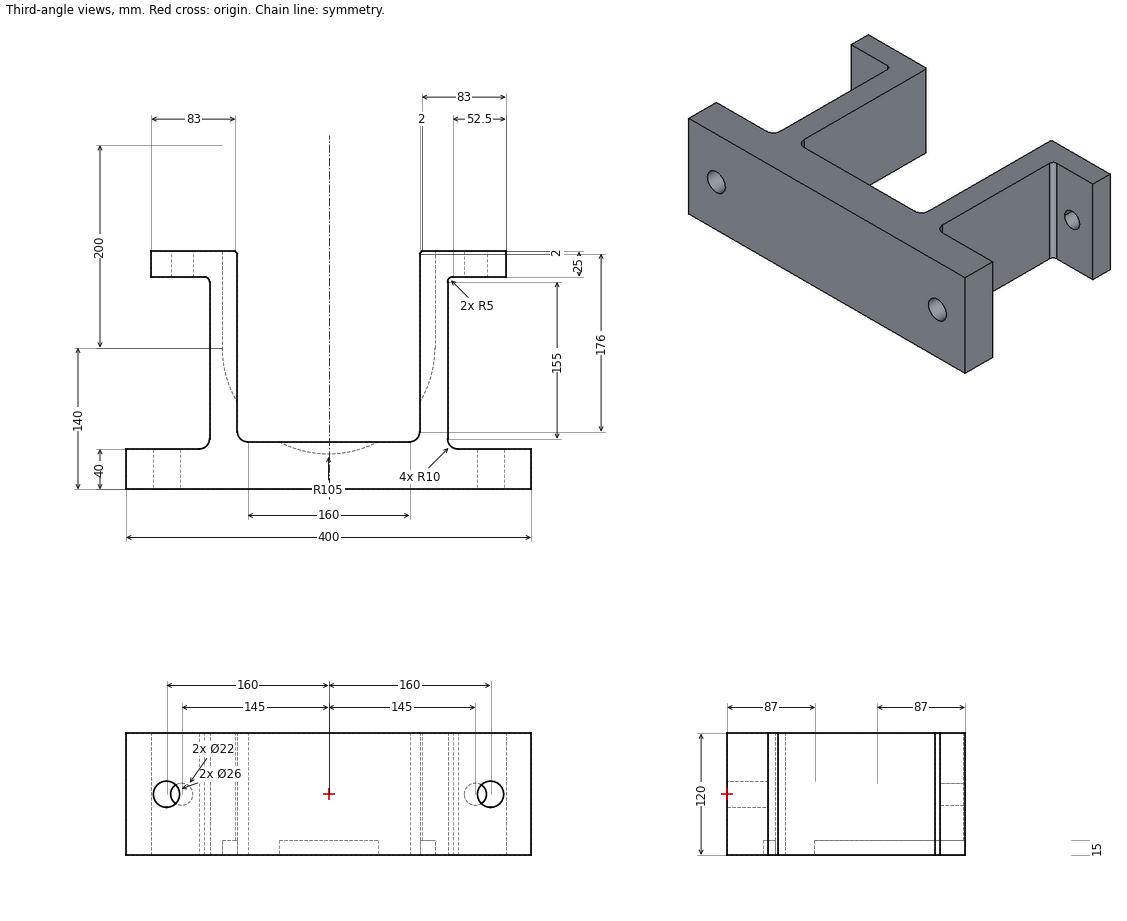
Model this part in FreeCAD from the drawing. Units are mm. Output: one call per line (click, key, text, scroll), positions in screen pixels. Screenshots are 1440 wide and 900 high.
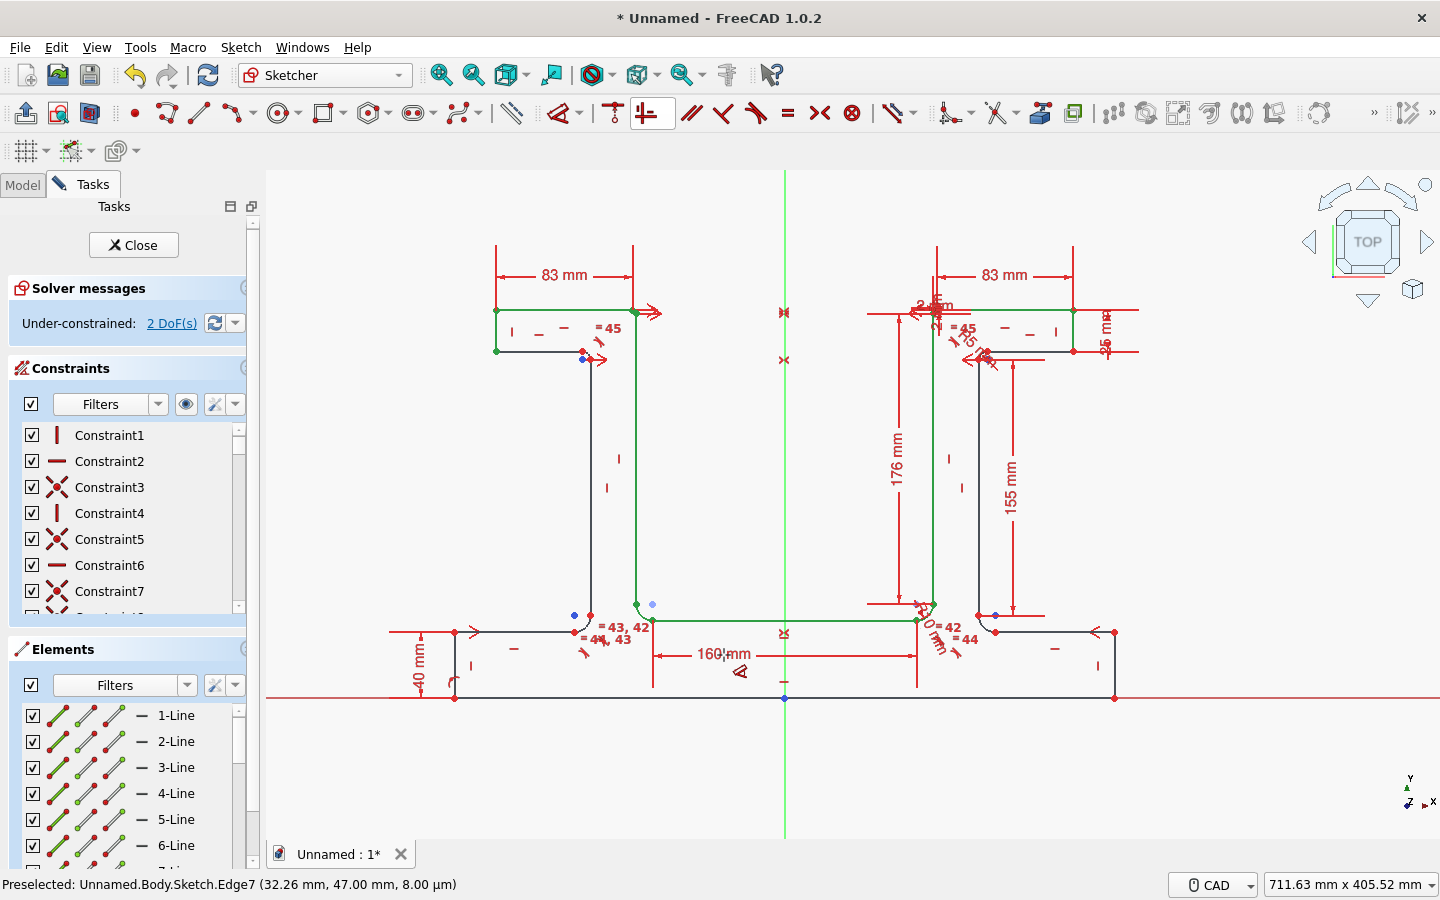
click(653, 698)
click(633, 732)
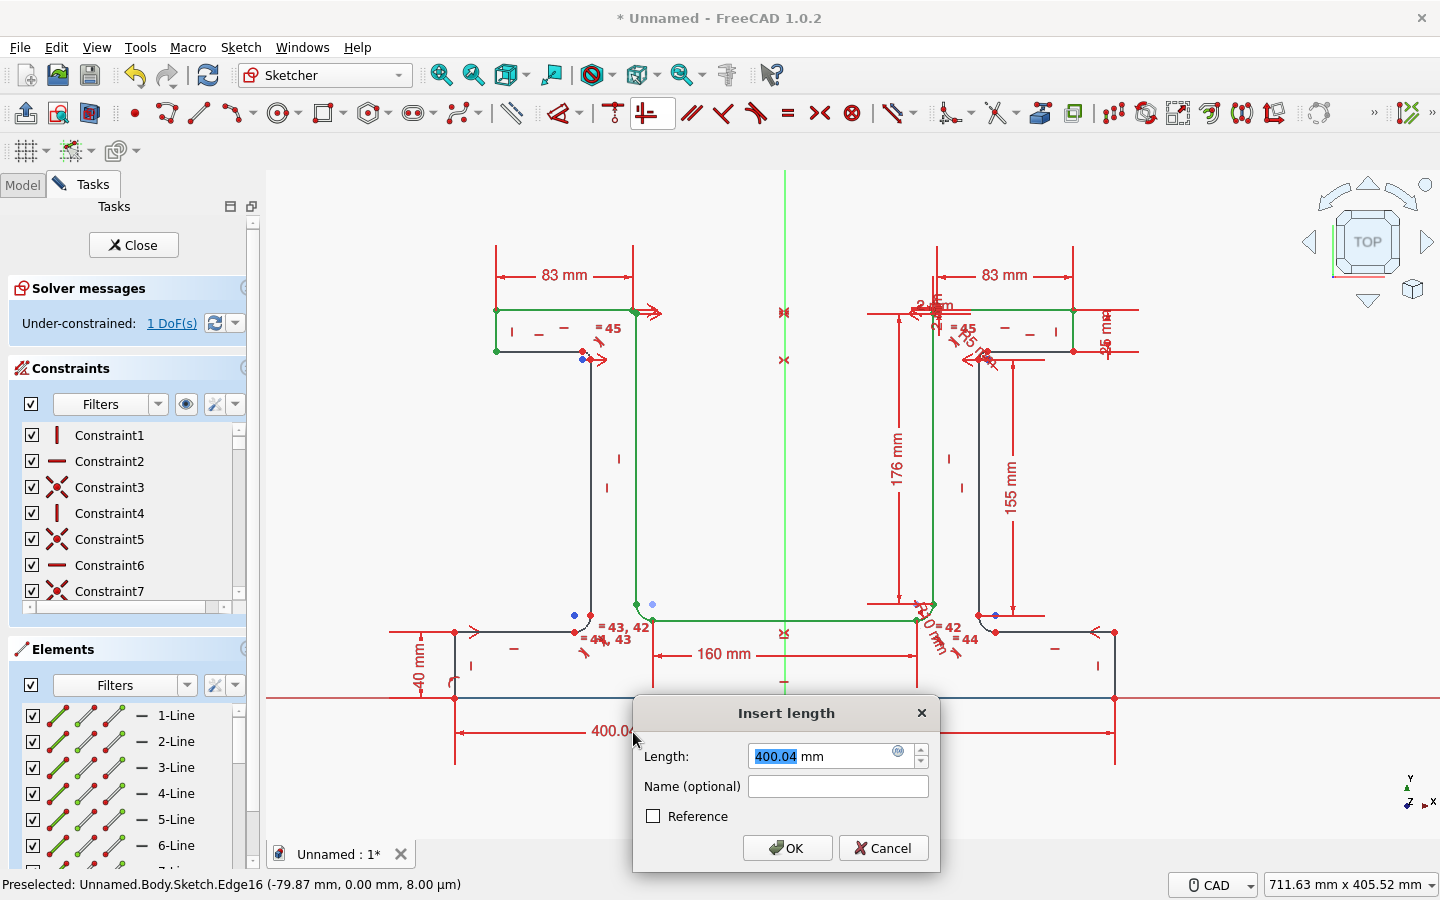
text(400)
key(Return)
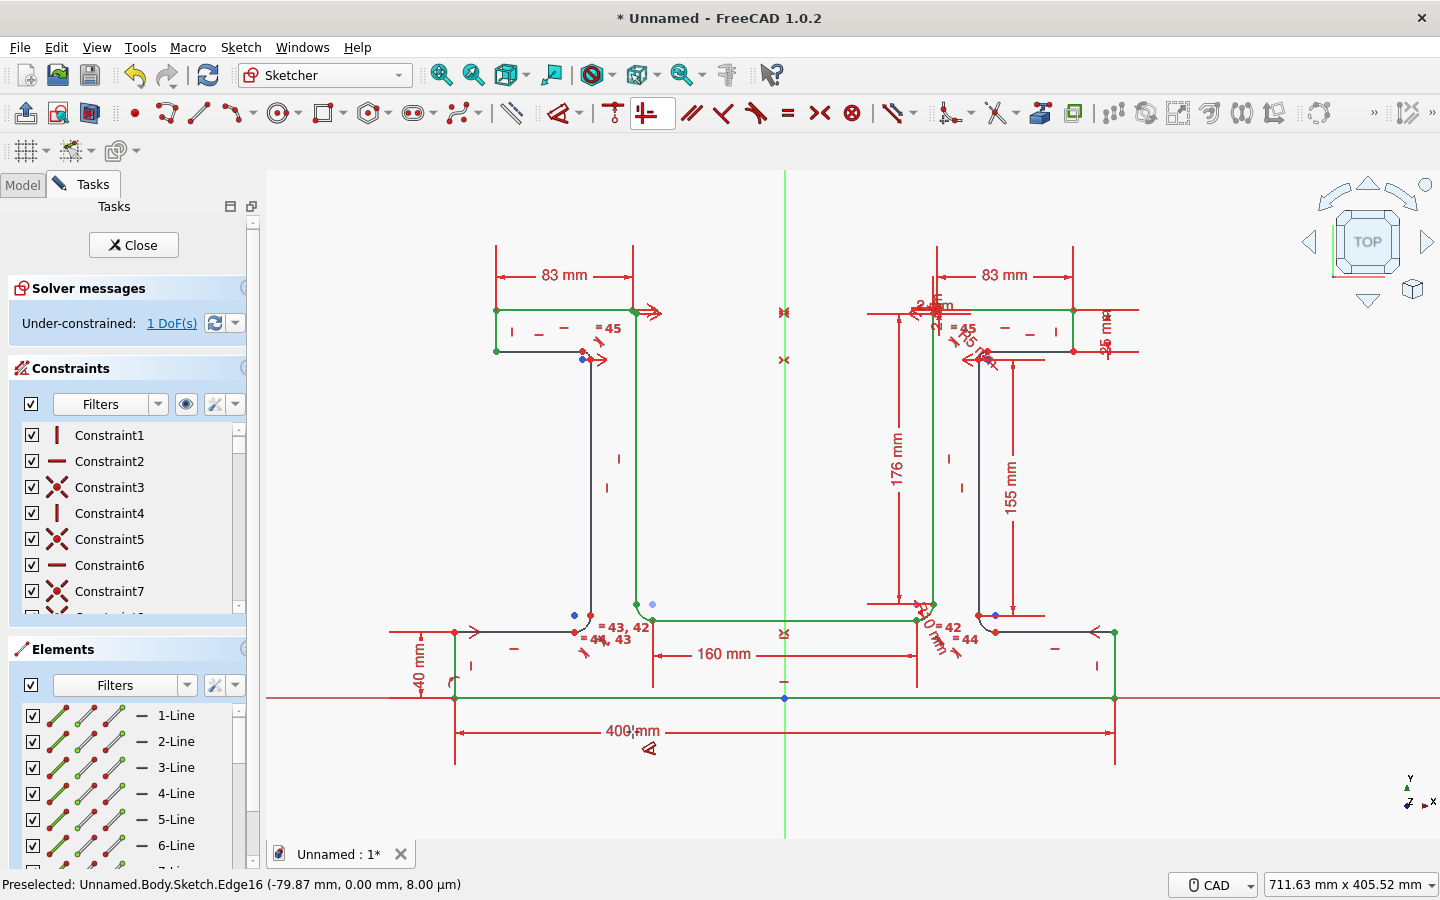
click(1013, 352)
click(1030, 386)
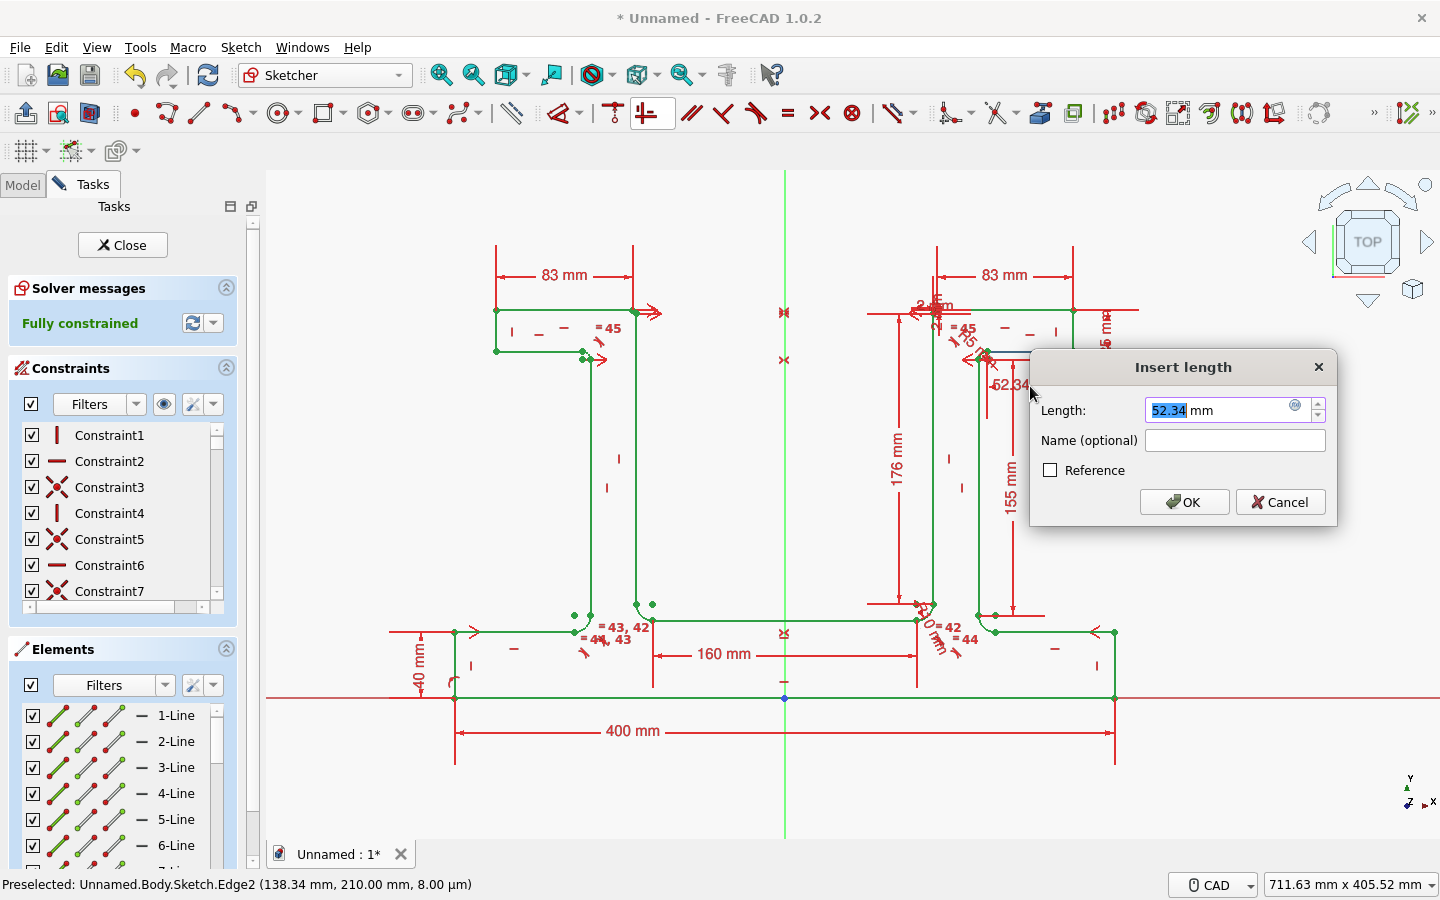
text(52.5)
key(Return)
key(Escape)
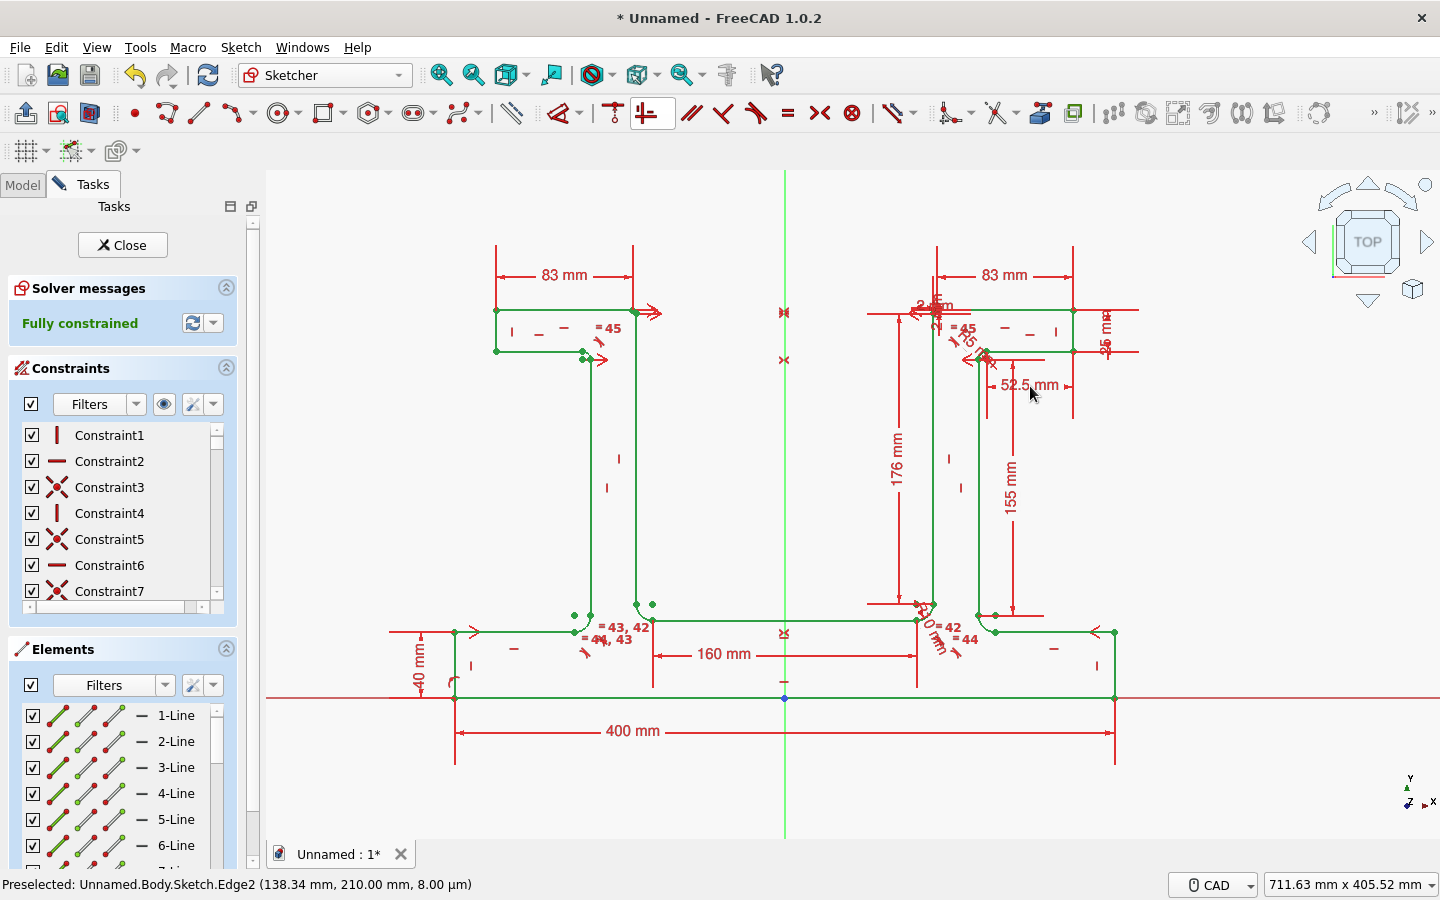
click(123, 245)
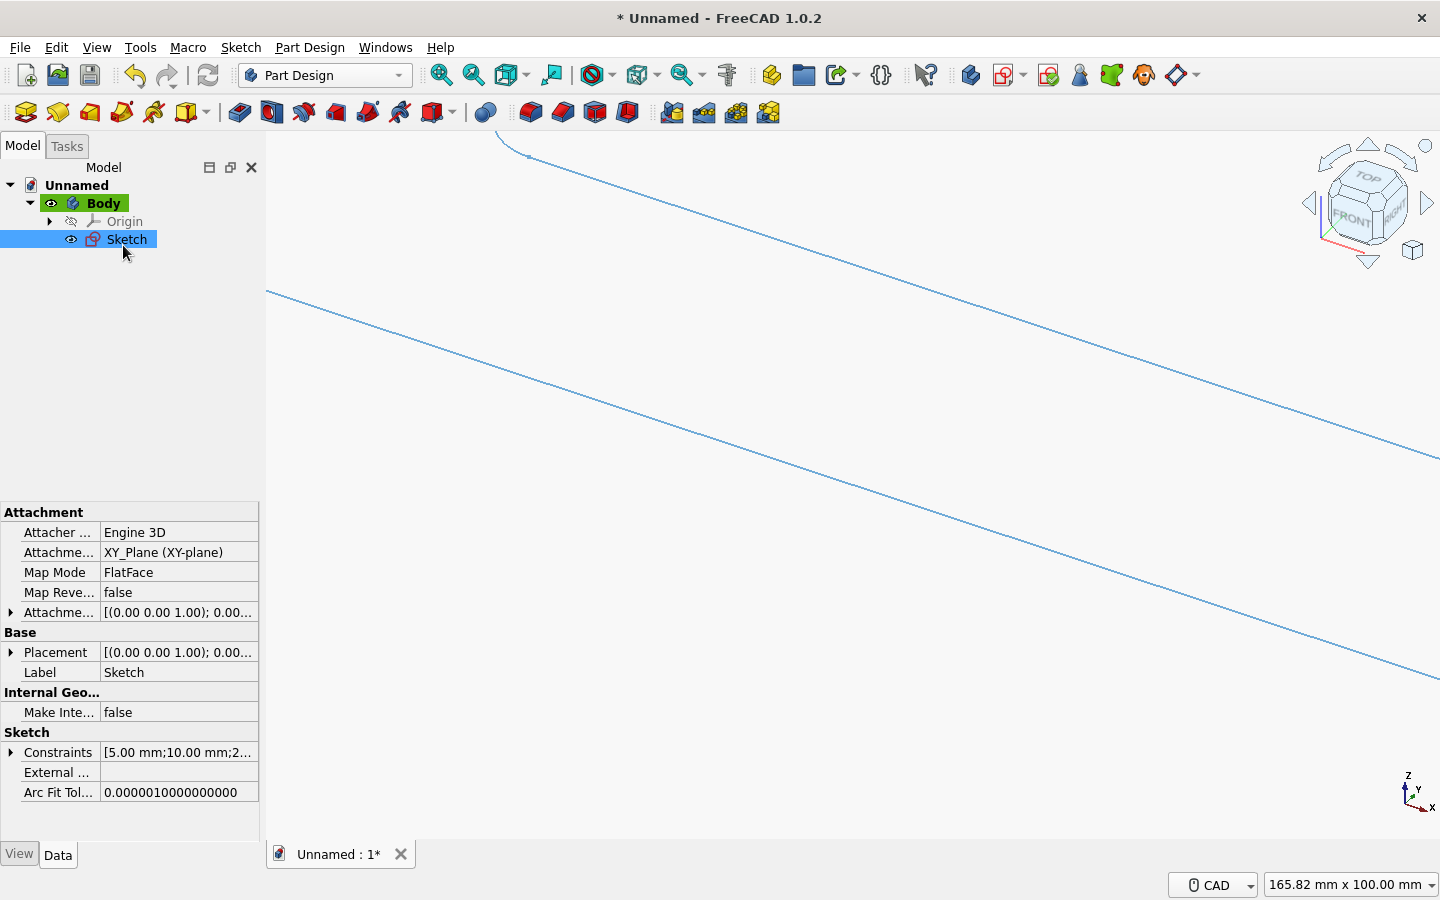
click(26, 112)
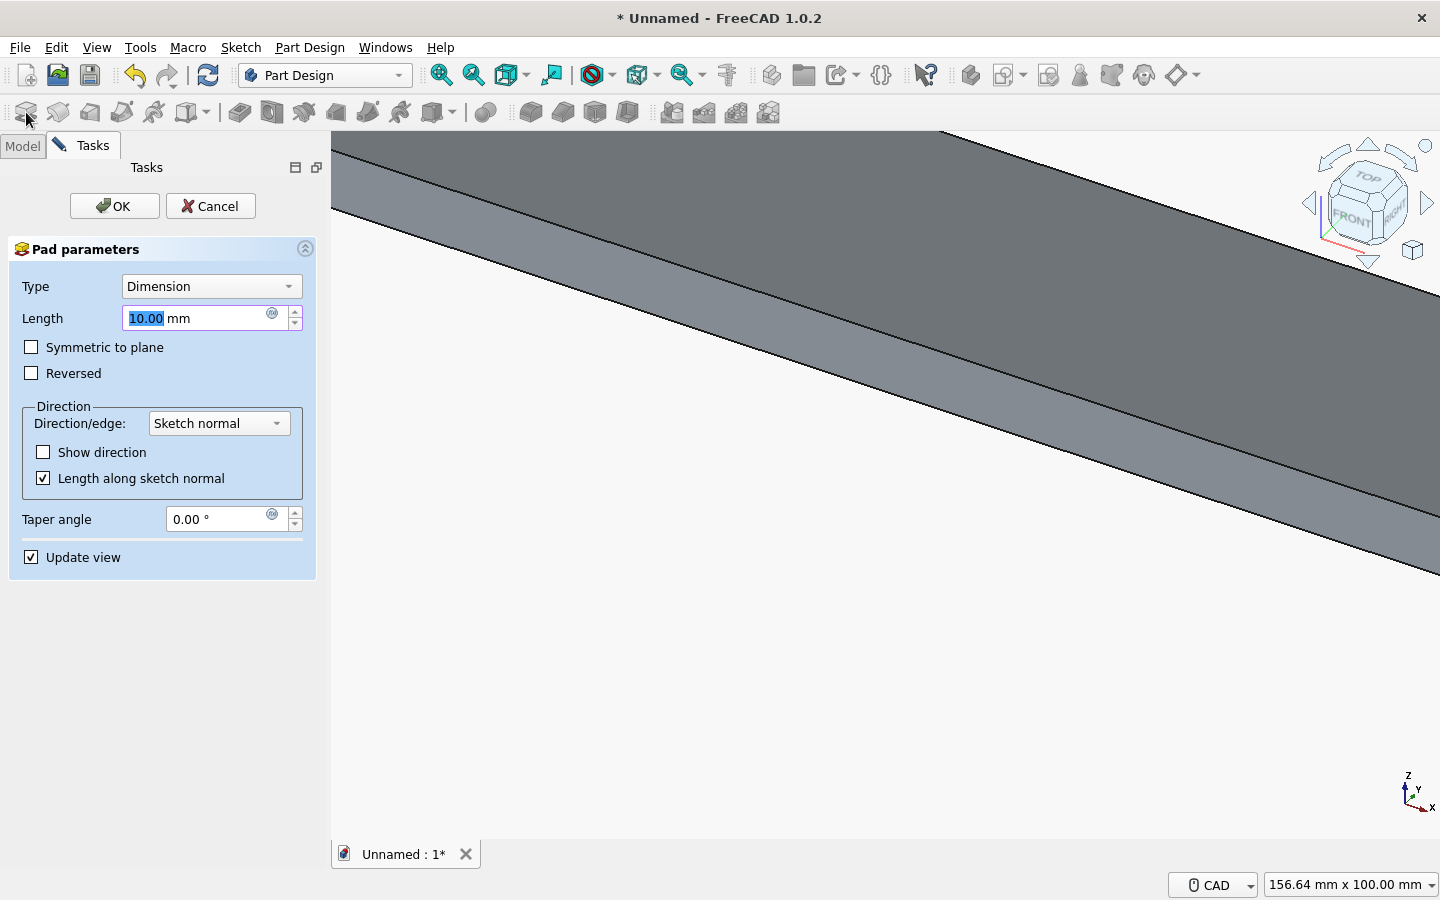
text(120)
key(Tab)